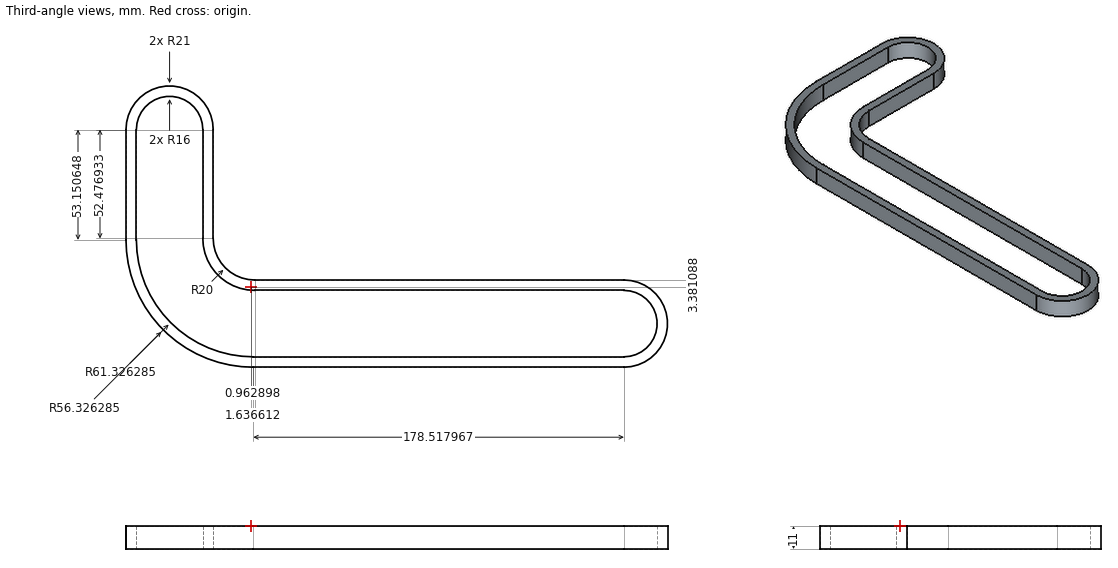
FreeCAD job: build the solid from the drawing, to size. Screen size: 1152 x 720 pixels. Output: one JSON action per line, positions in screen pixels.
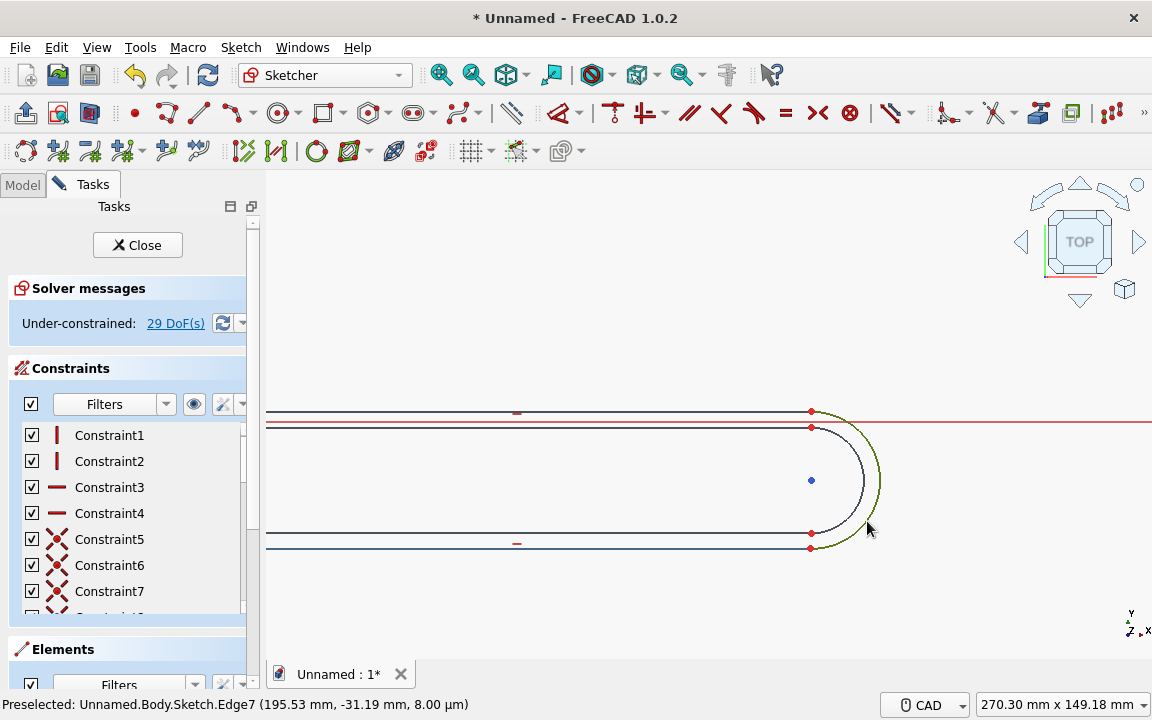
{"action": "left_click", "coordinate": [754, 114]}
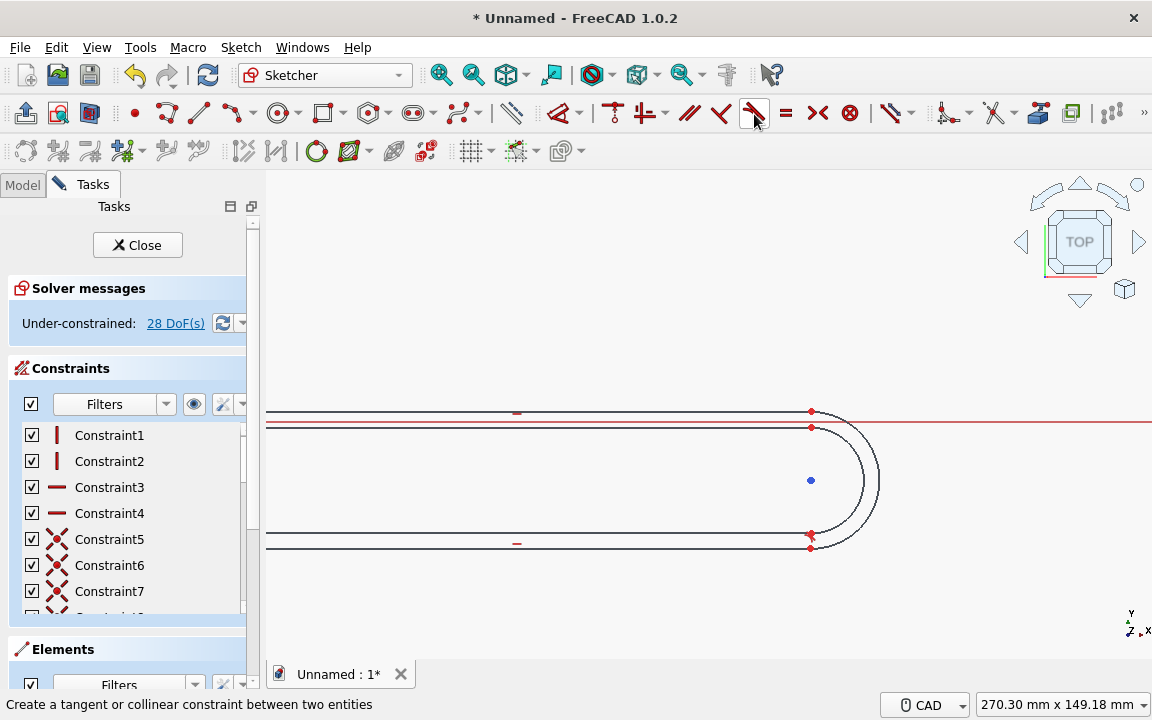
{"action": "scroll", "coordinate": [637, 412], "scroll_direction": "up", "scroll_amount": 2}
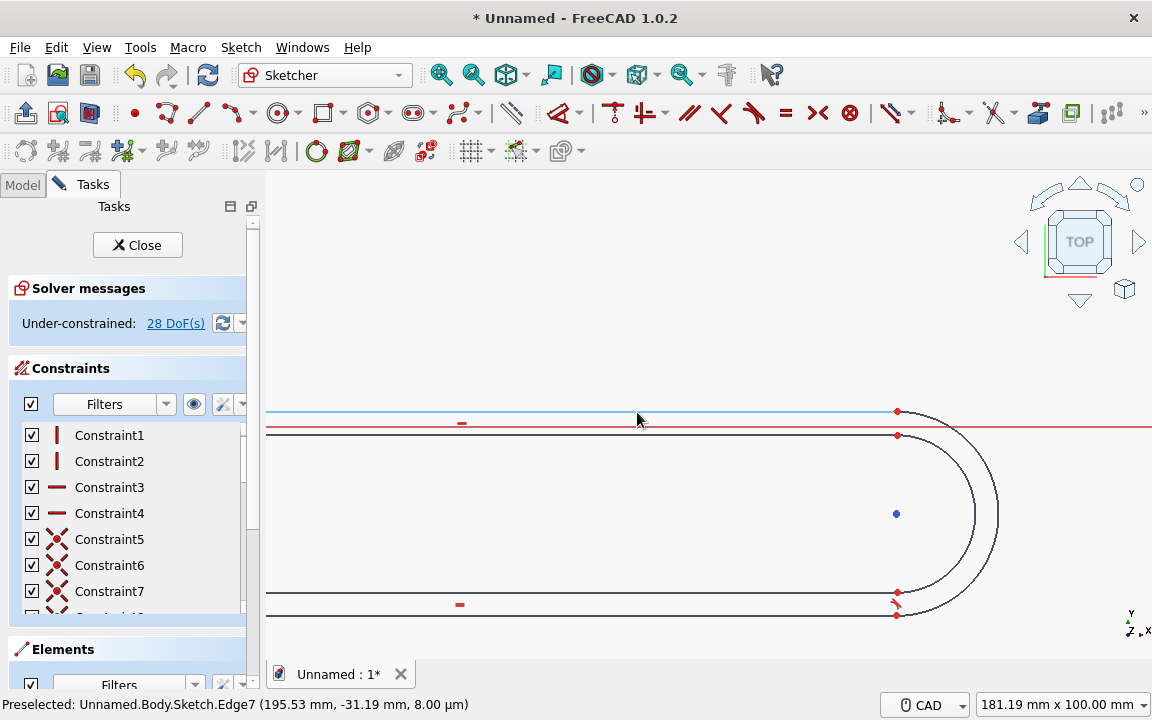
{"action": "left_click", "coordinate": [636, 412]}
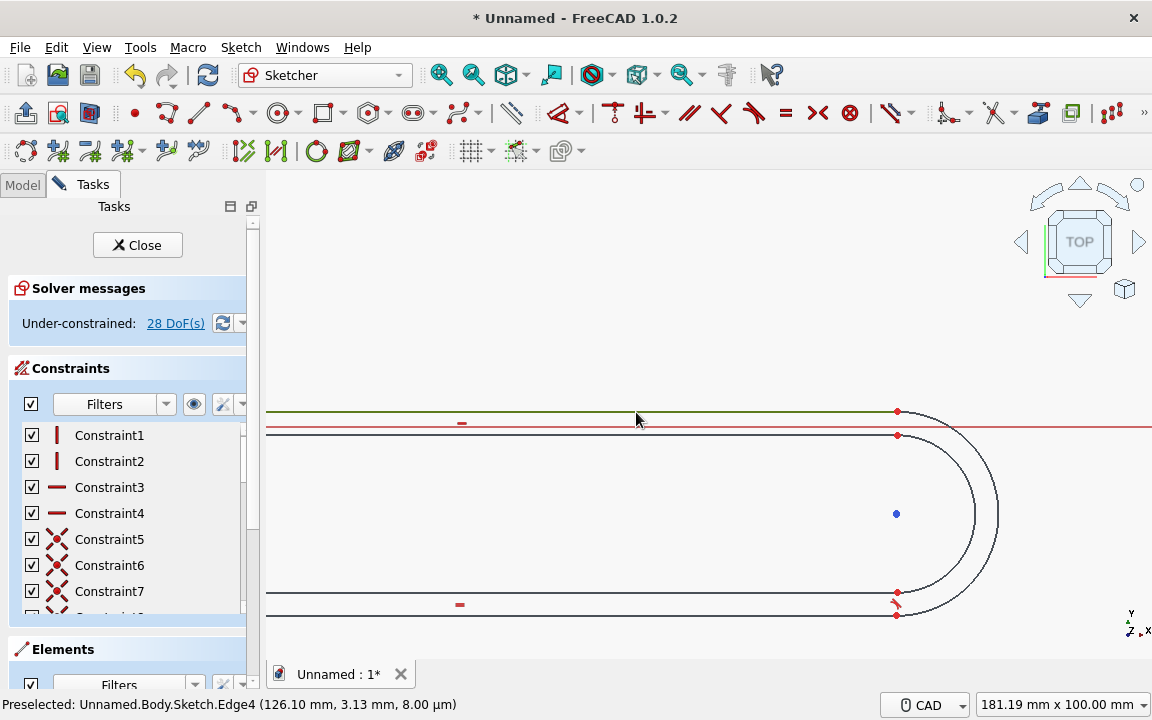
{"action": "left_click", "coordinate": [979, 574]}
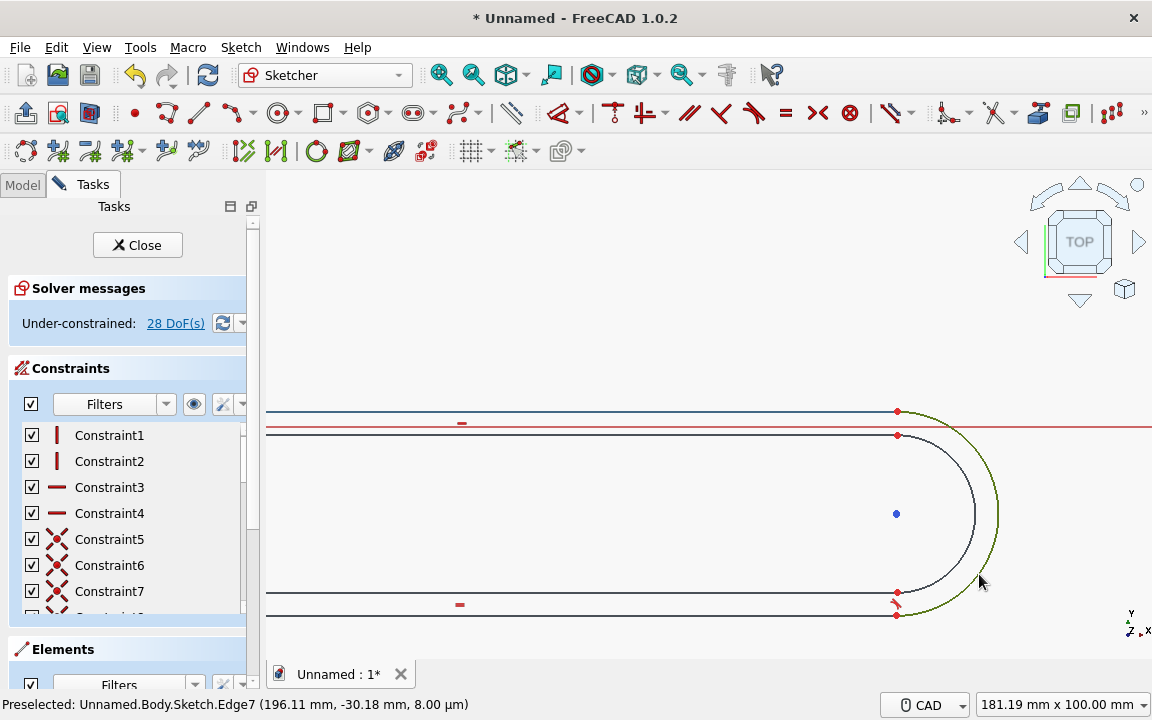
{"action": "key", "text": "t"}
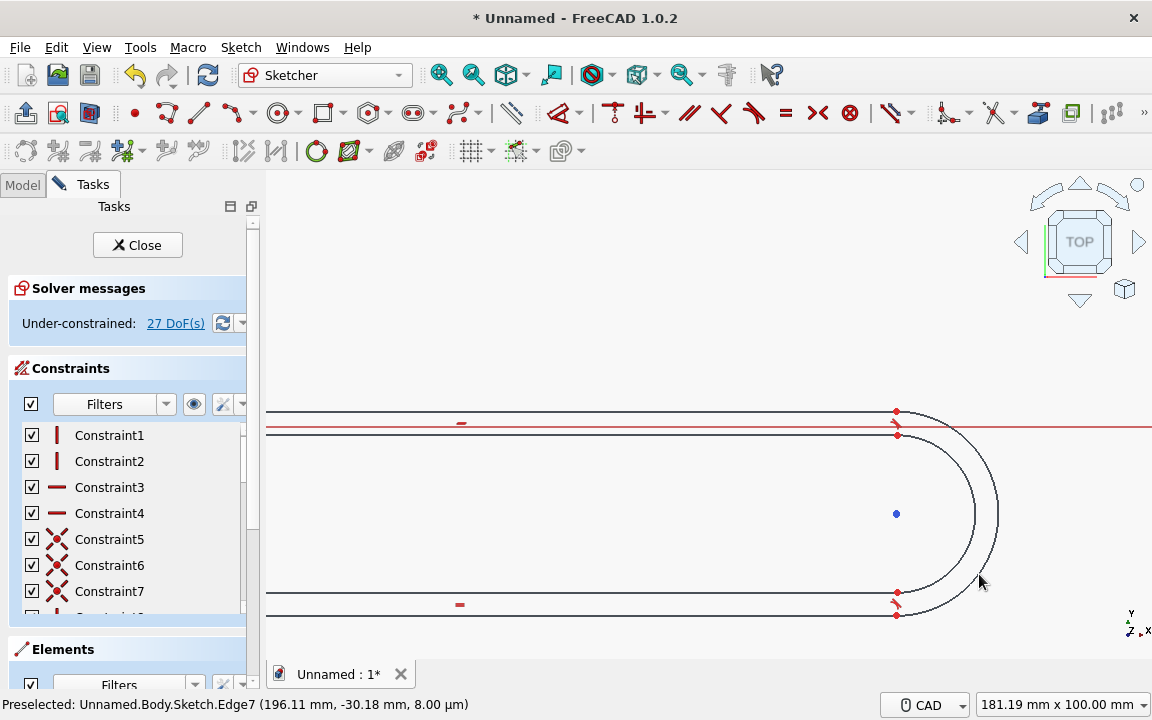
{"action": "left_click", "coordinate": [636, 412]}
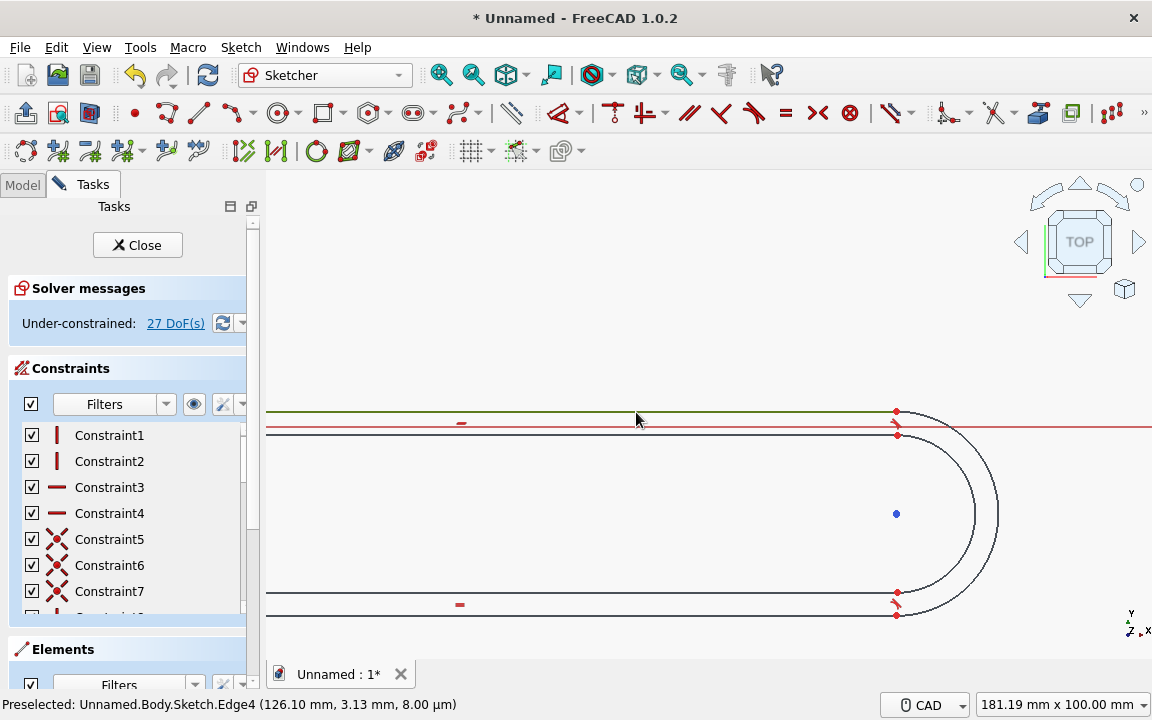
{"action": "scroll", "coordinate": [803, 490], "scroll_direction": "down", "scroll_amount": 5}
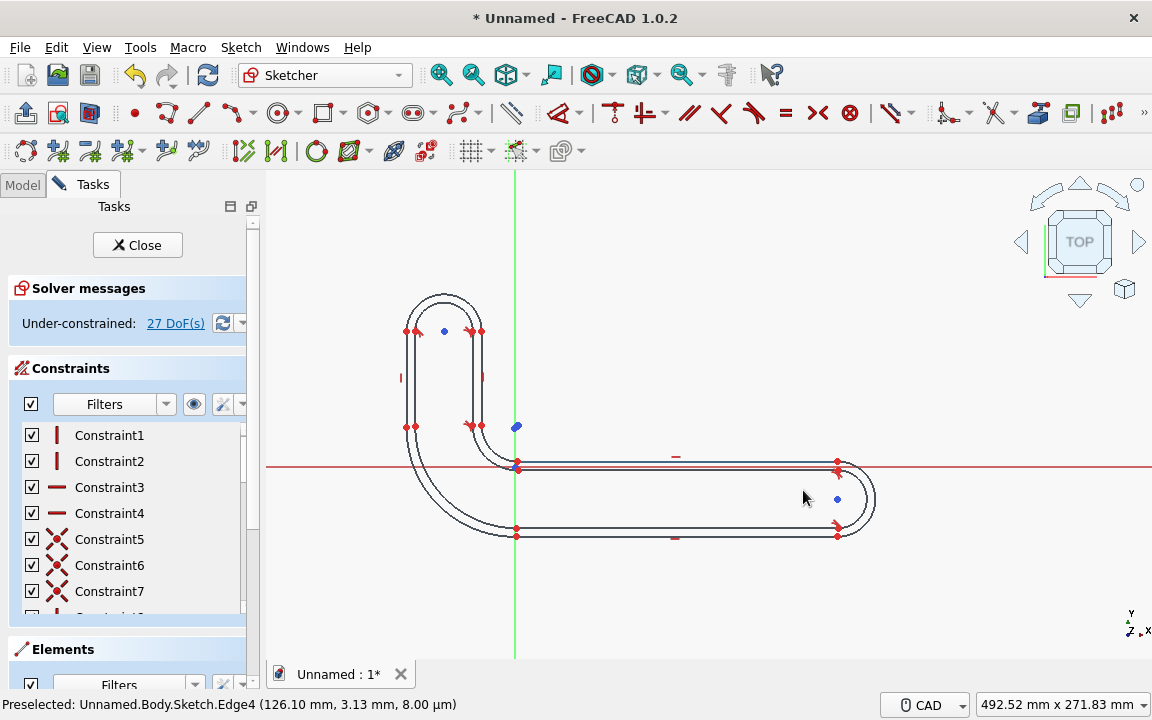
{"action": "scroll", "coordinate": [486, 442], "scroll_direction": "up", "scroll_amount": 3}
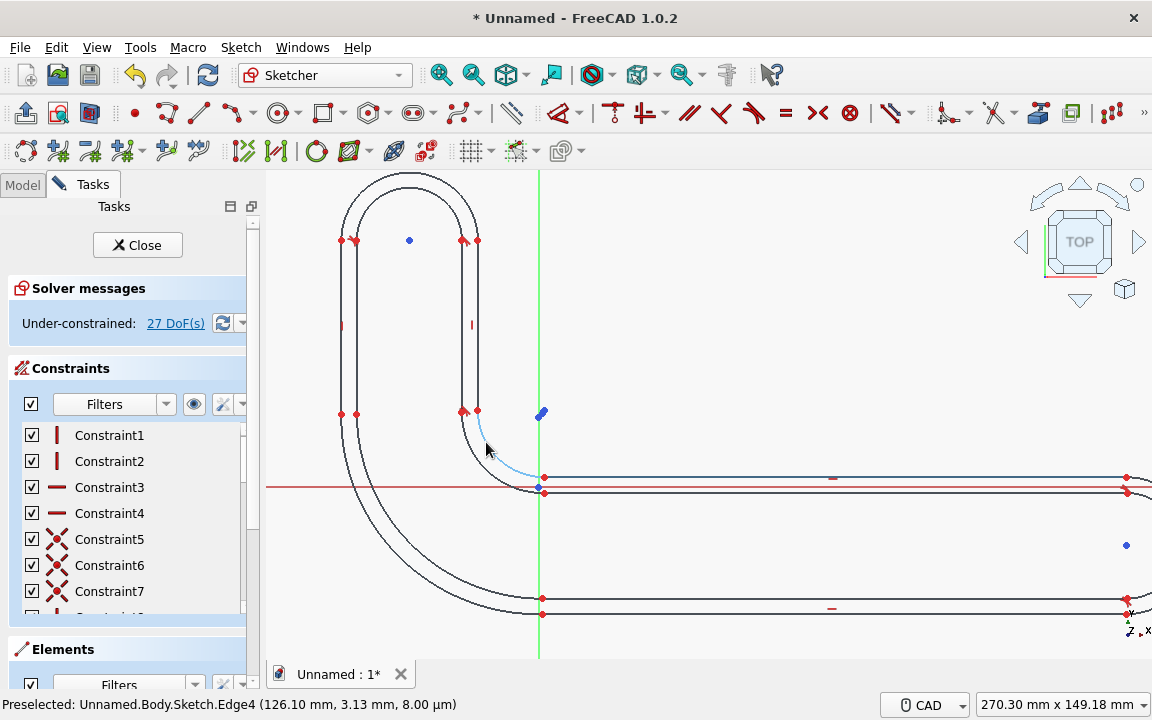
{"action": "left_click", "coordinate": [485, 441]}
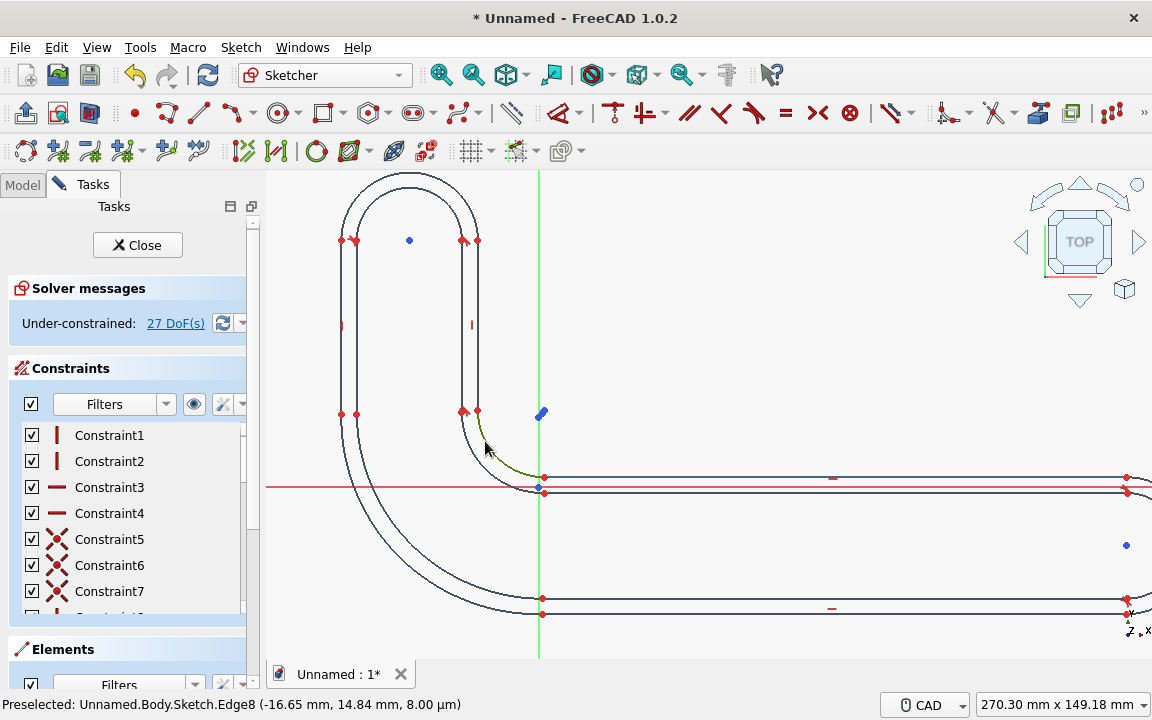
{"action": "left_click", "coordinate": [754, 114]}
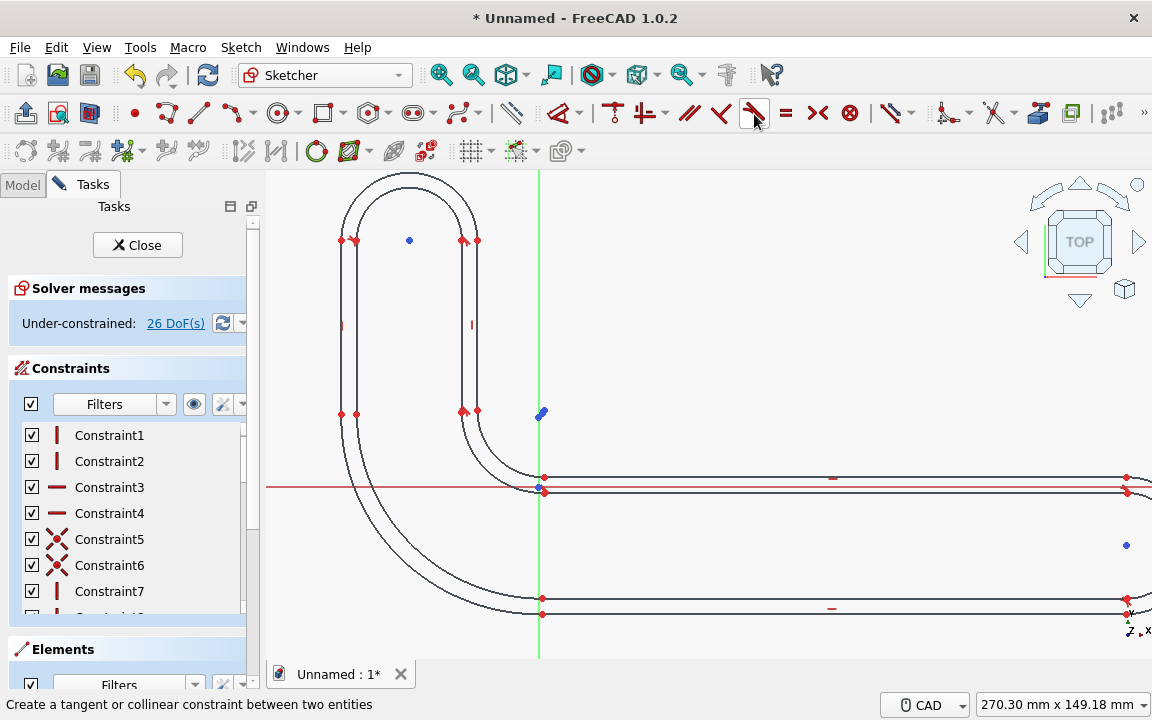
{"action": "left_click", "coordinate": [357, 362]}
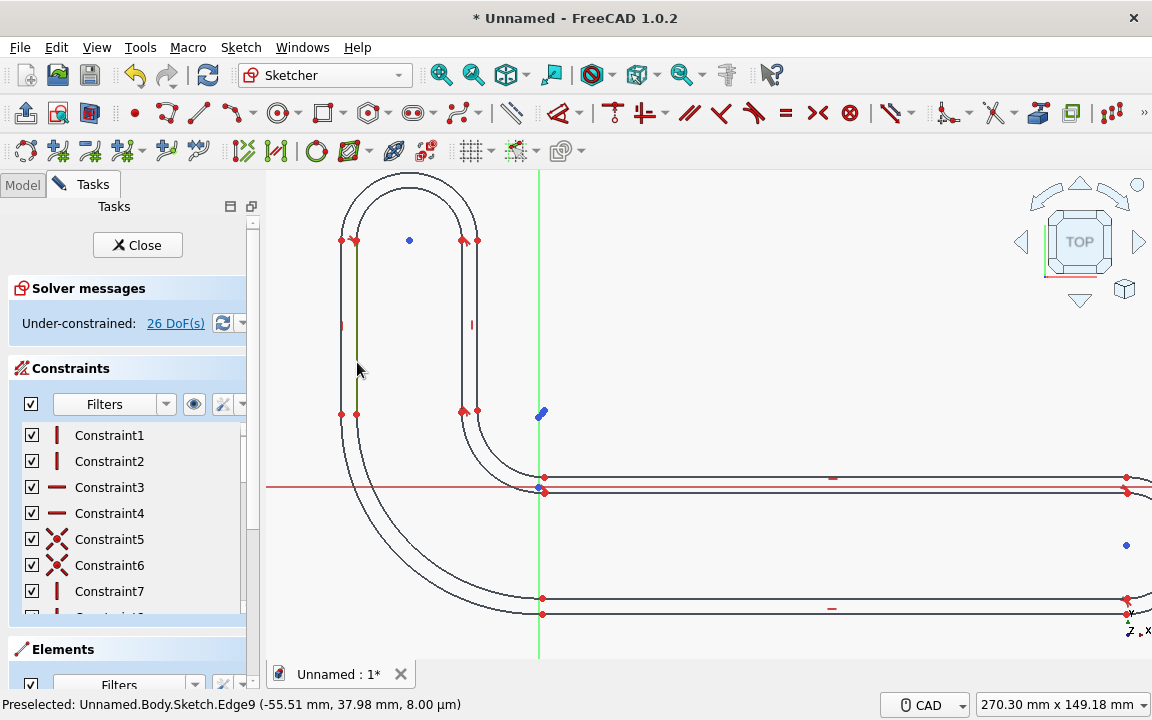
{"action": "left_click", "coordinate": [452, 209]}